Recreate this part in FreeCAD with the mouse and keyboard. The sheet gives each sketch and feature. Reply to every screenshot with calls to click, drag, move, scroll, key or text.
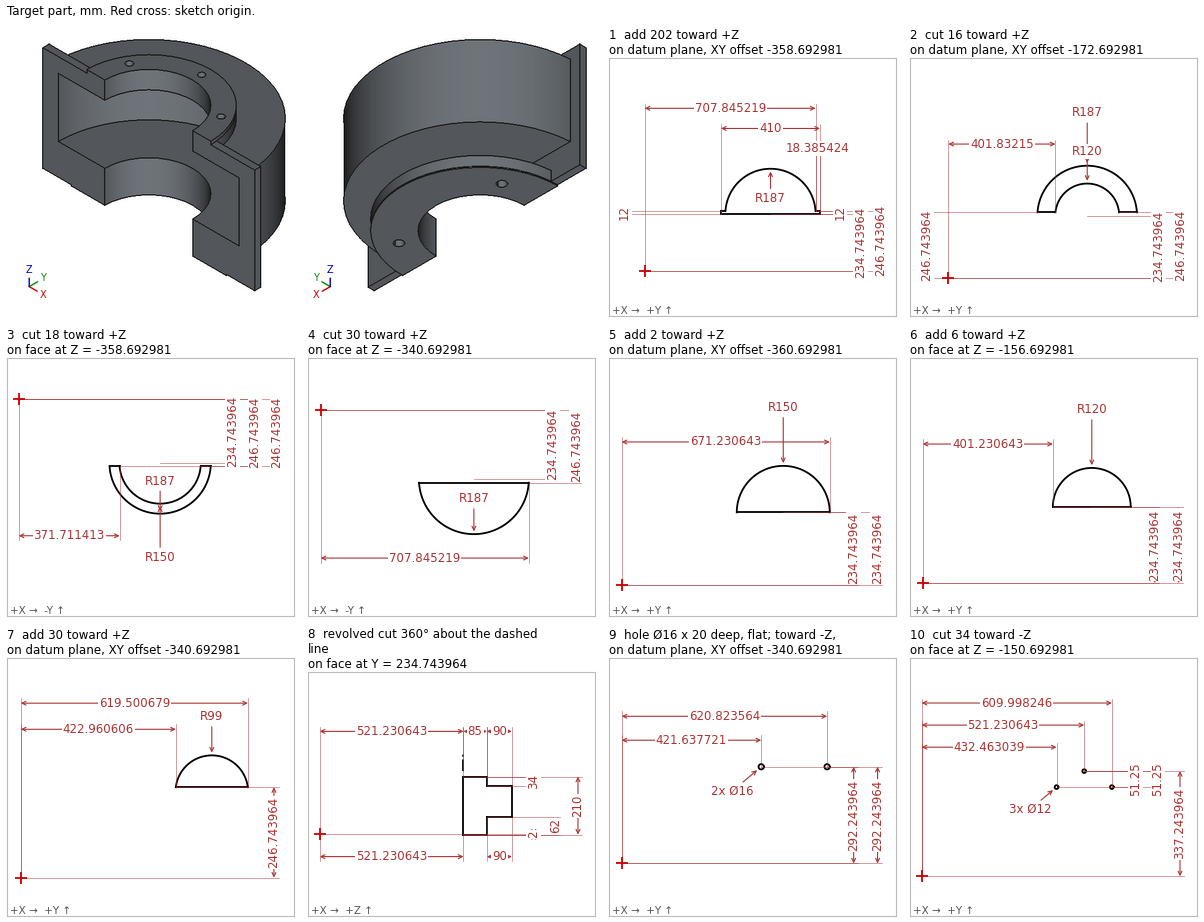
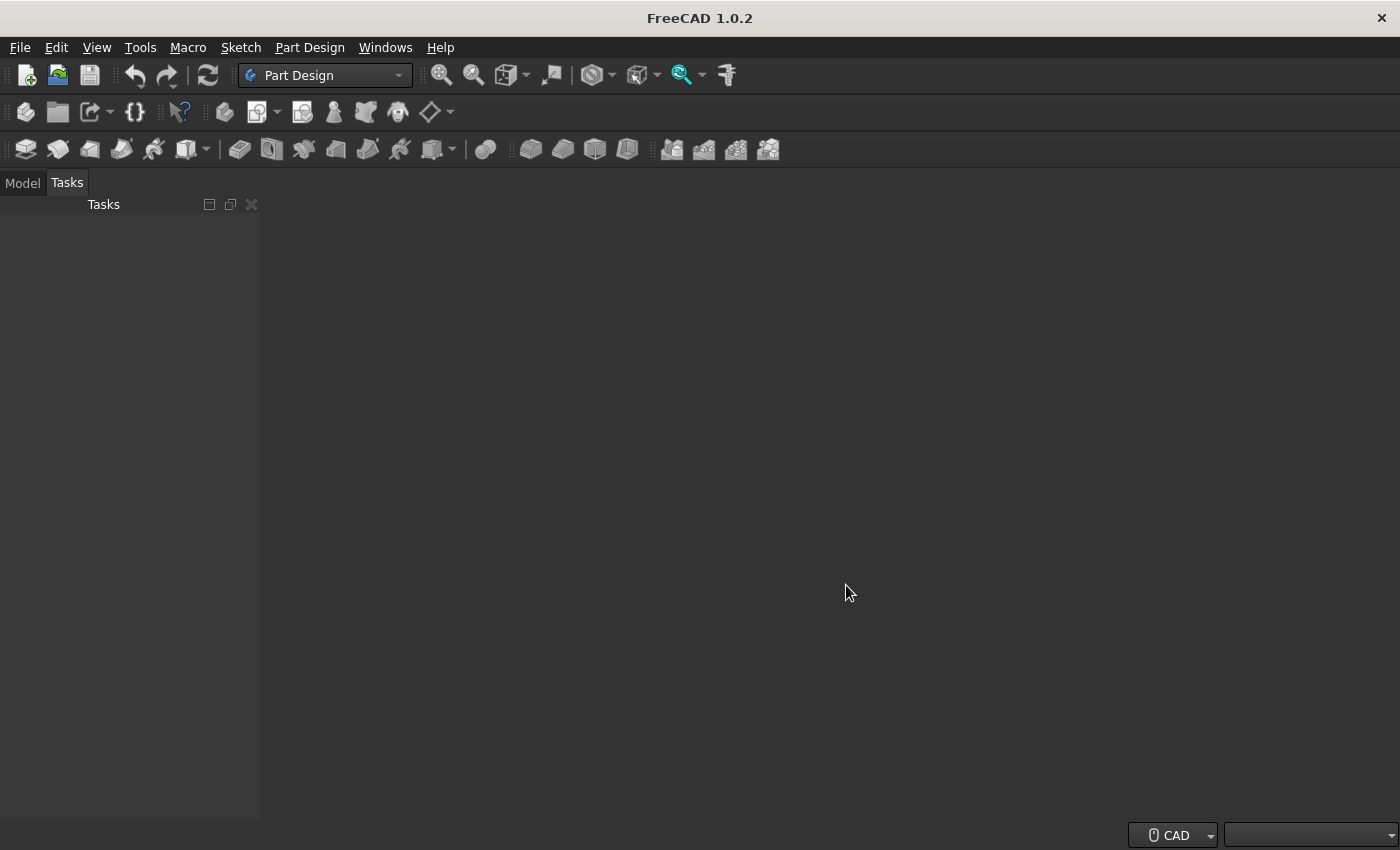
key(ctrl+n)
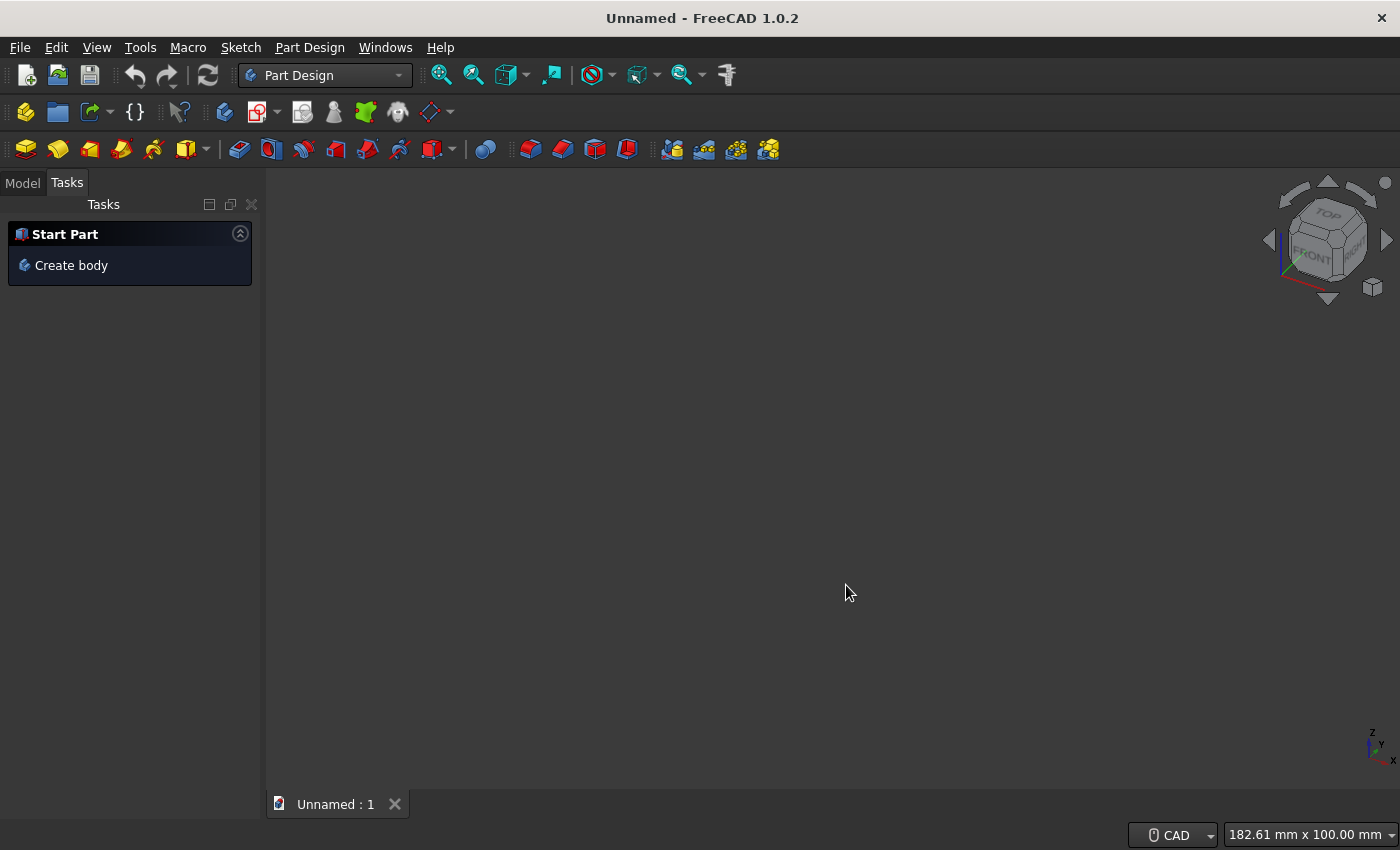
click(226, 112)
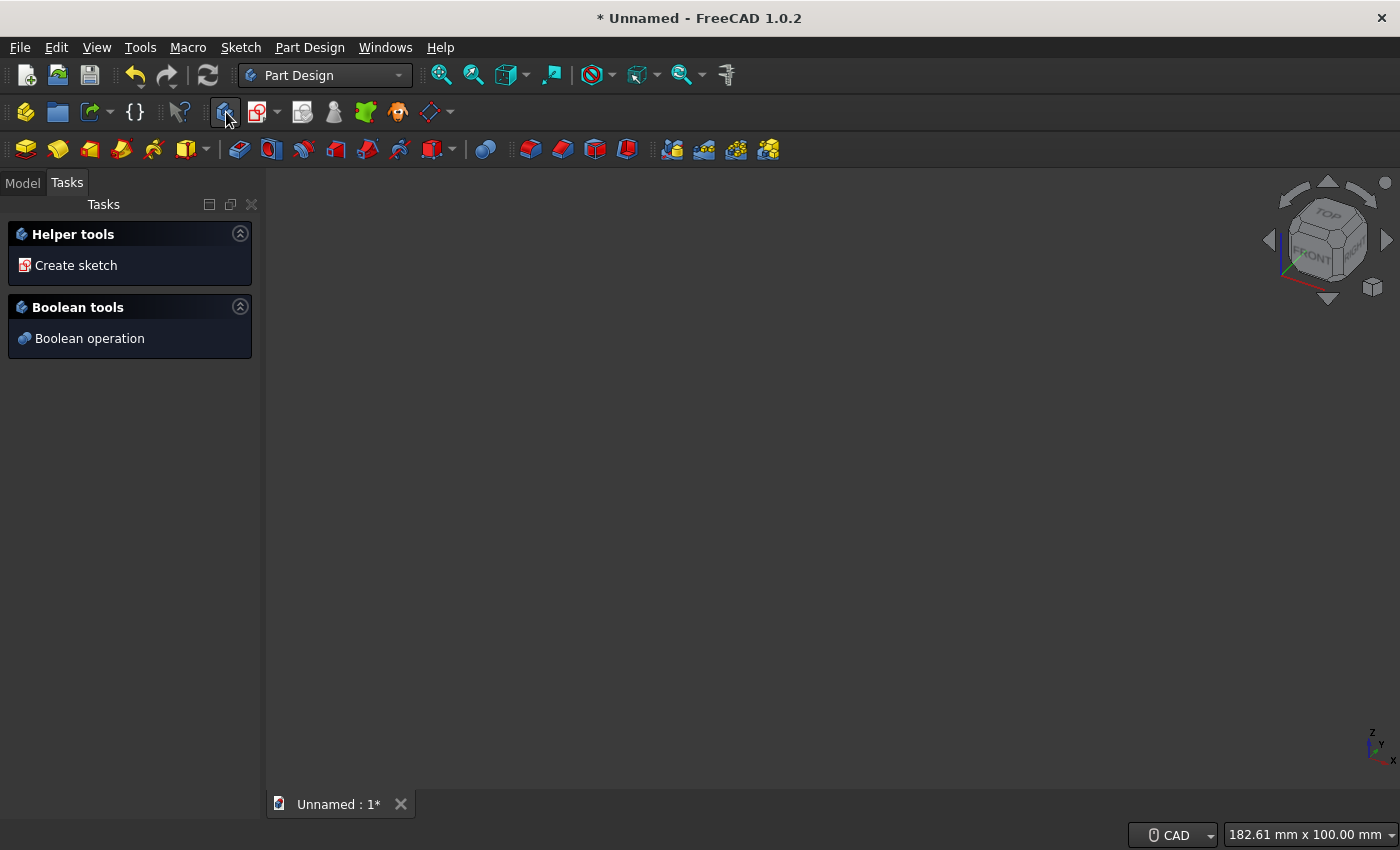
click(23, 182)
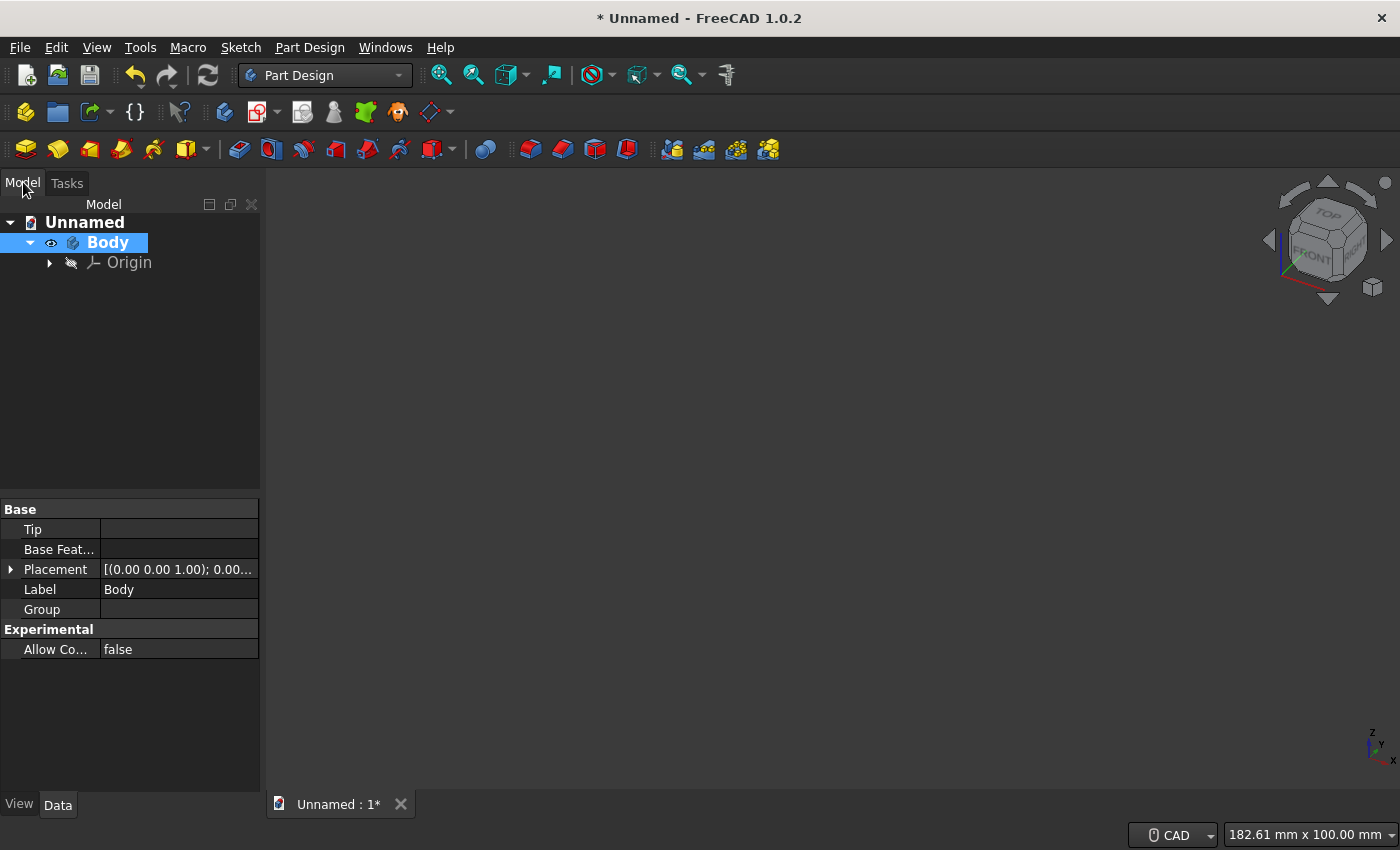
click(50, 263)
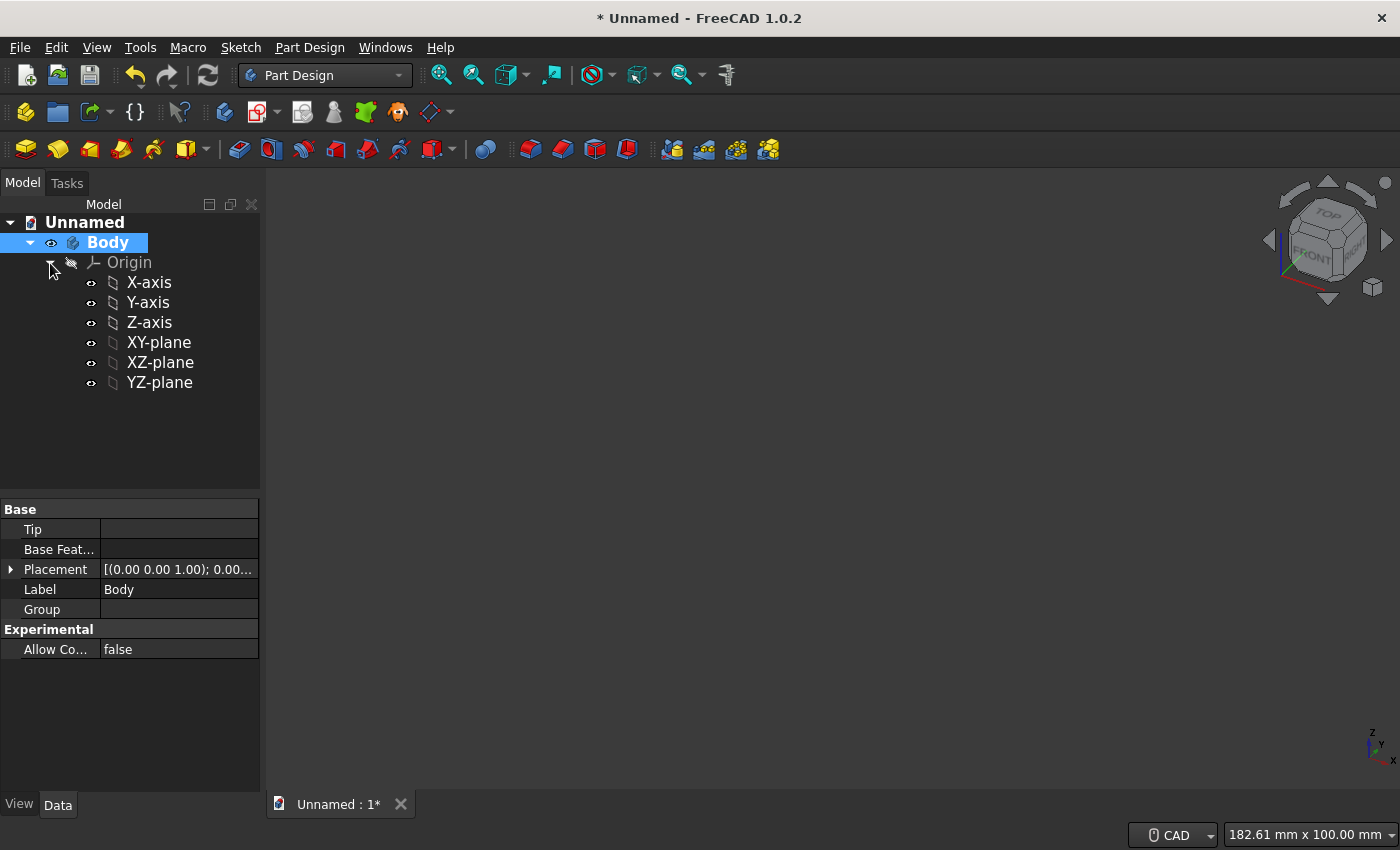
click(136, 343)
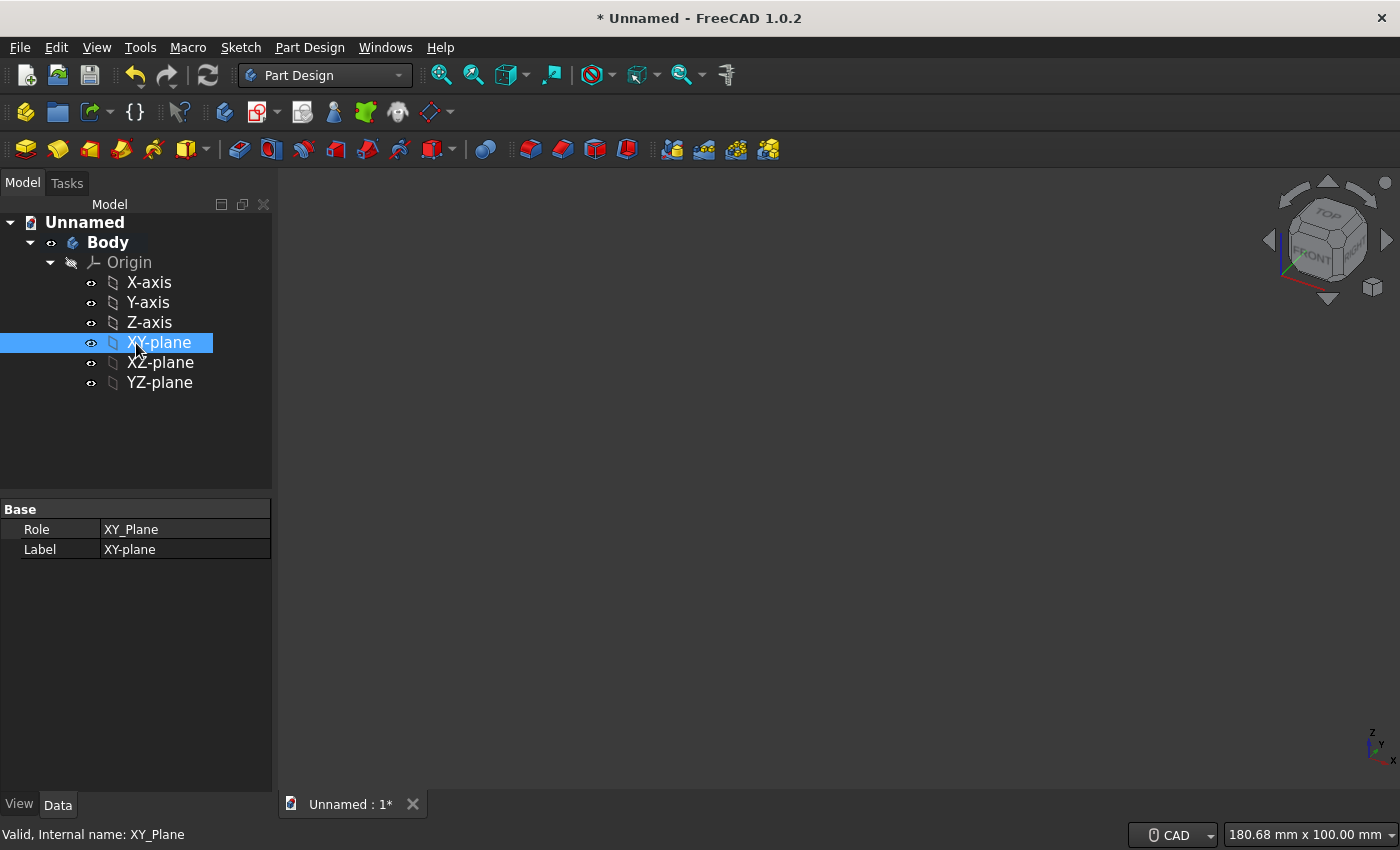
click(430, 112)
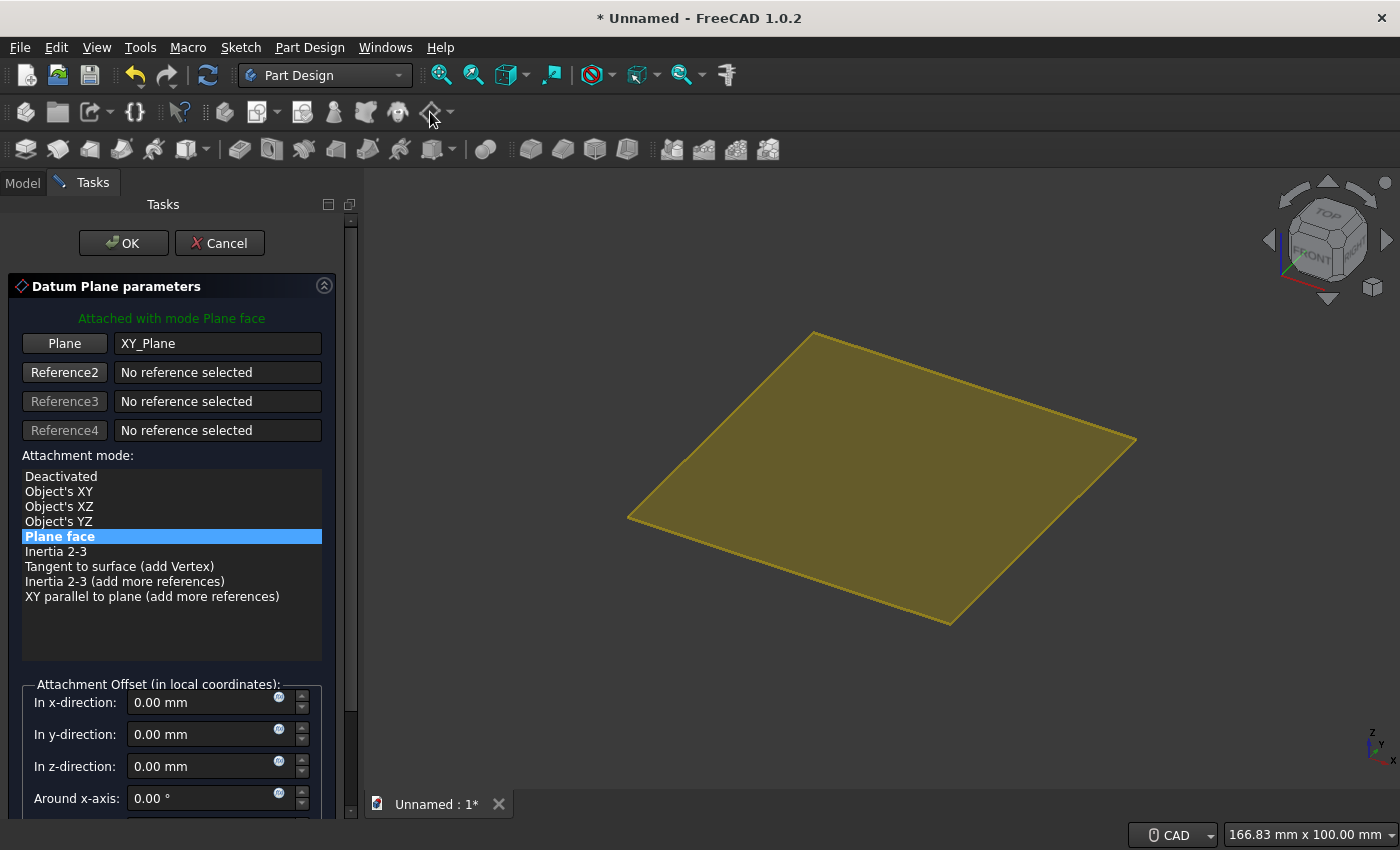
triple_click(210, 766)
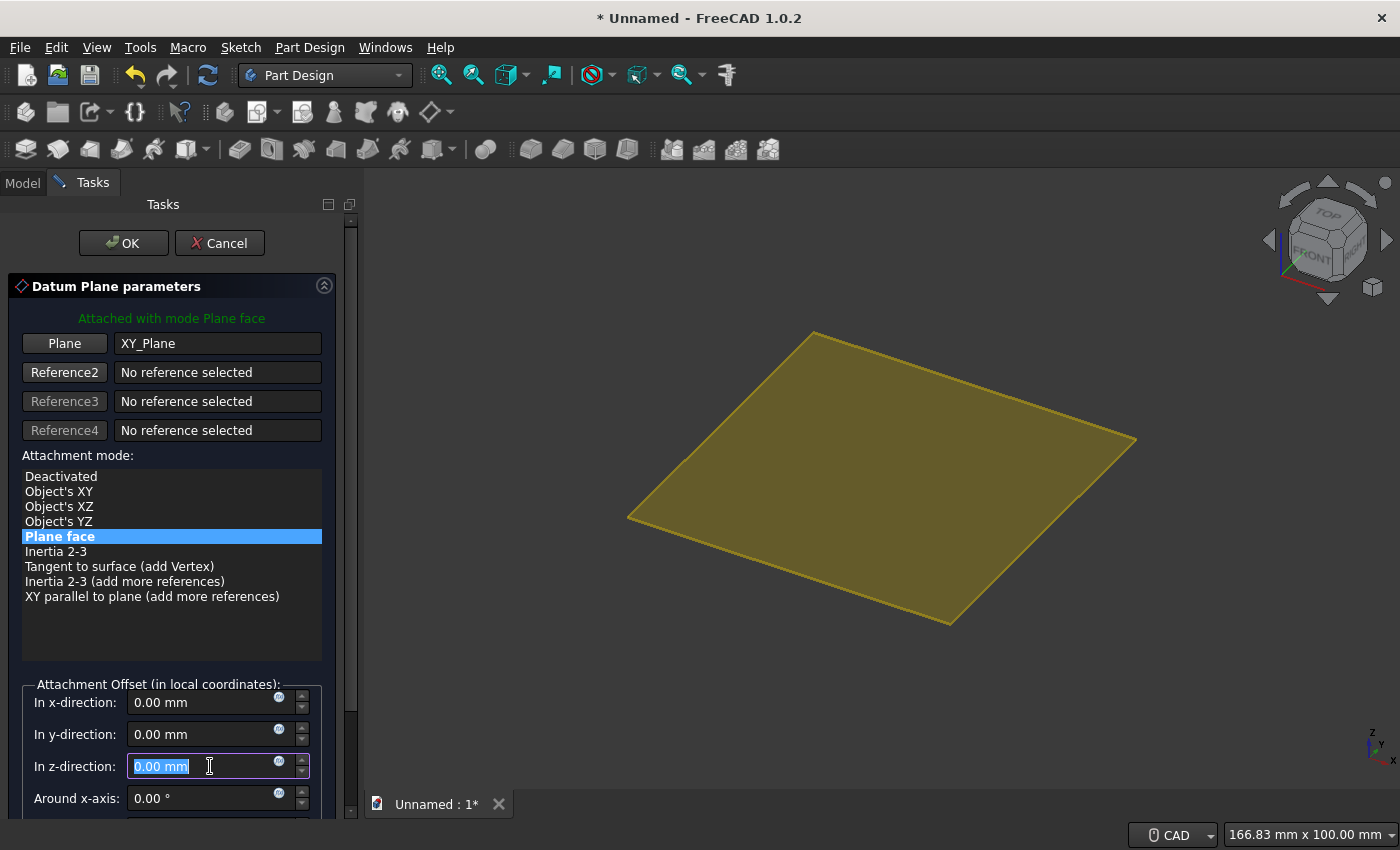
text(-358.692981)
key(Tab)